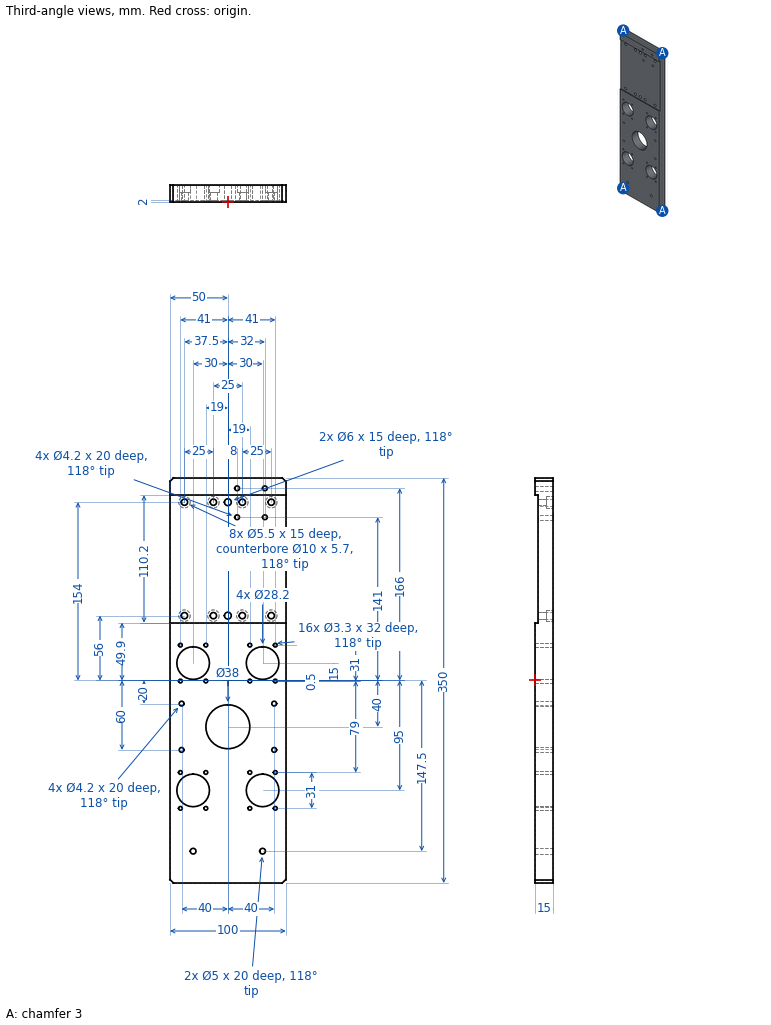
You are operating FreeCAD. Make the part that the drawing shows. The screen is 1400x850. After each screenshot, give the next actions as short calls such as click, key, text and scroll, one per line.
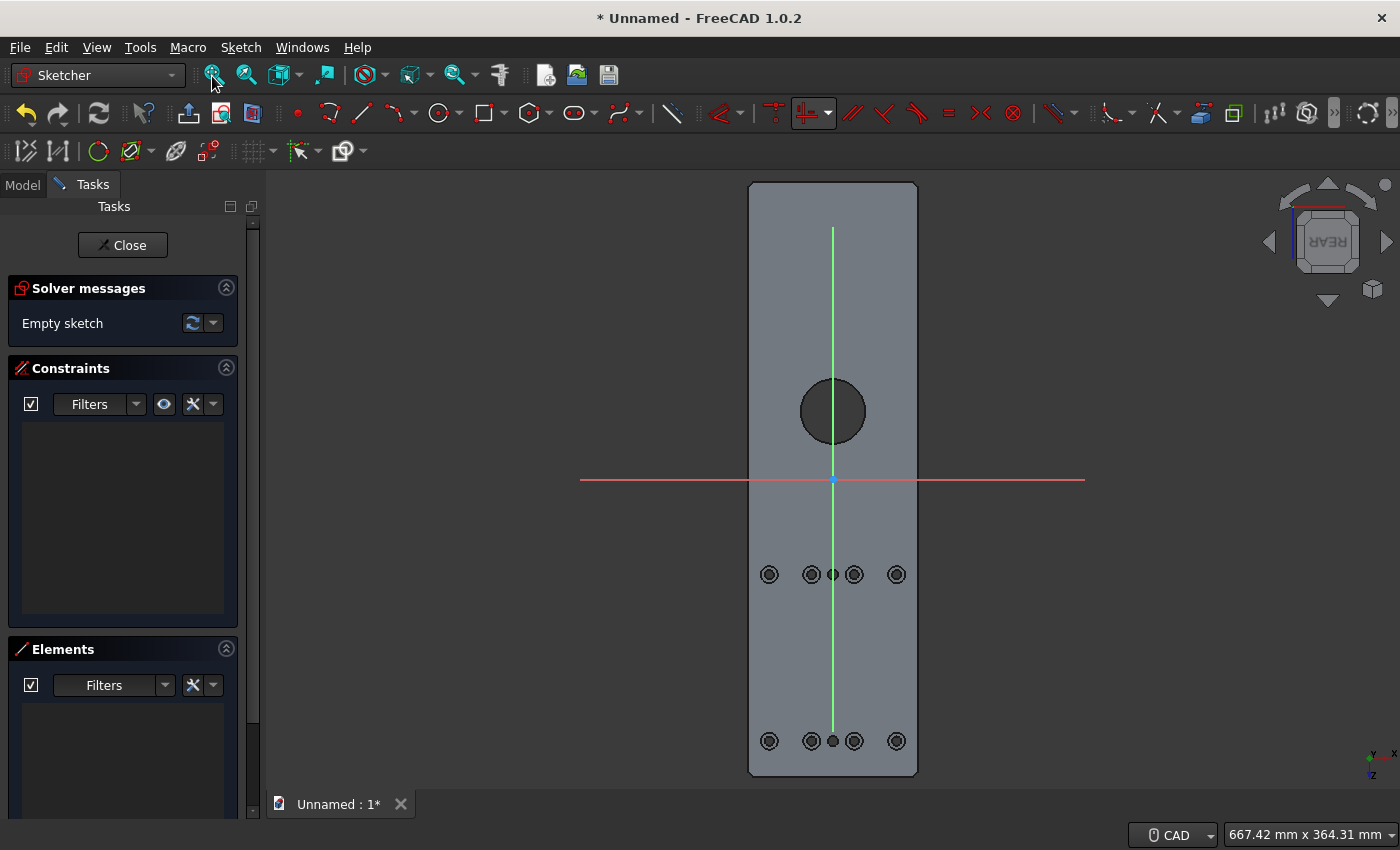
scroll(916, 329, up, 3)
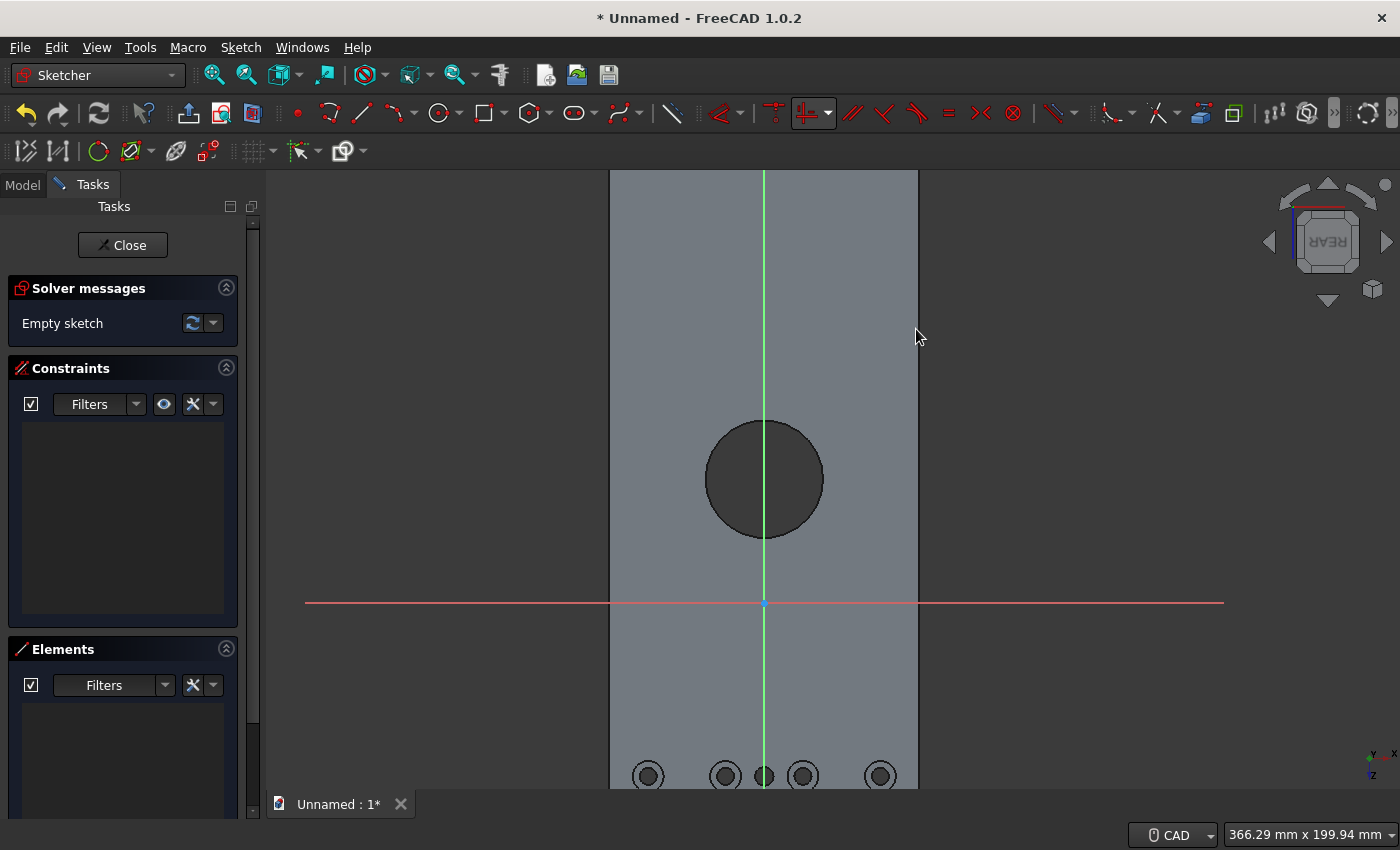
key(g)
key(c)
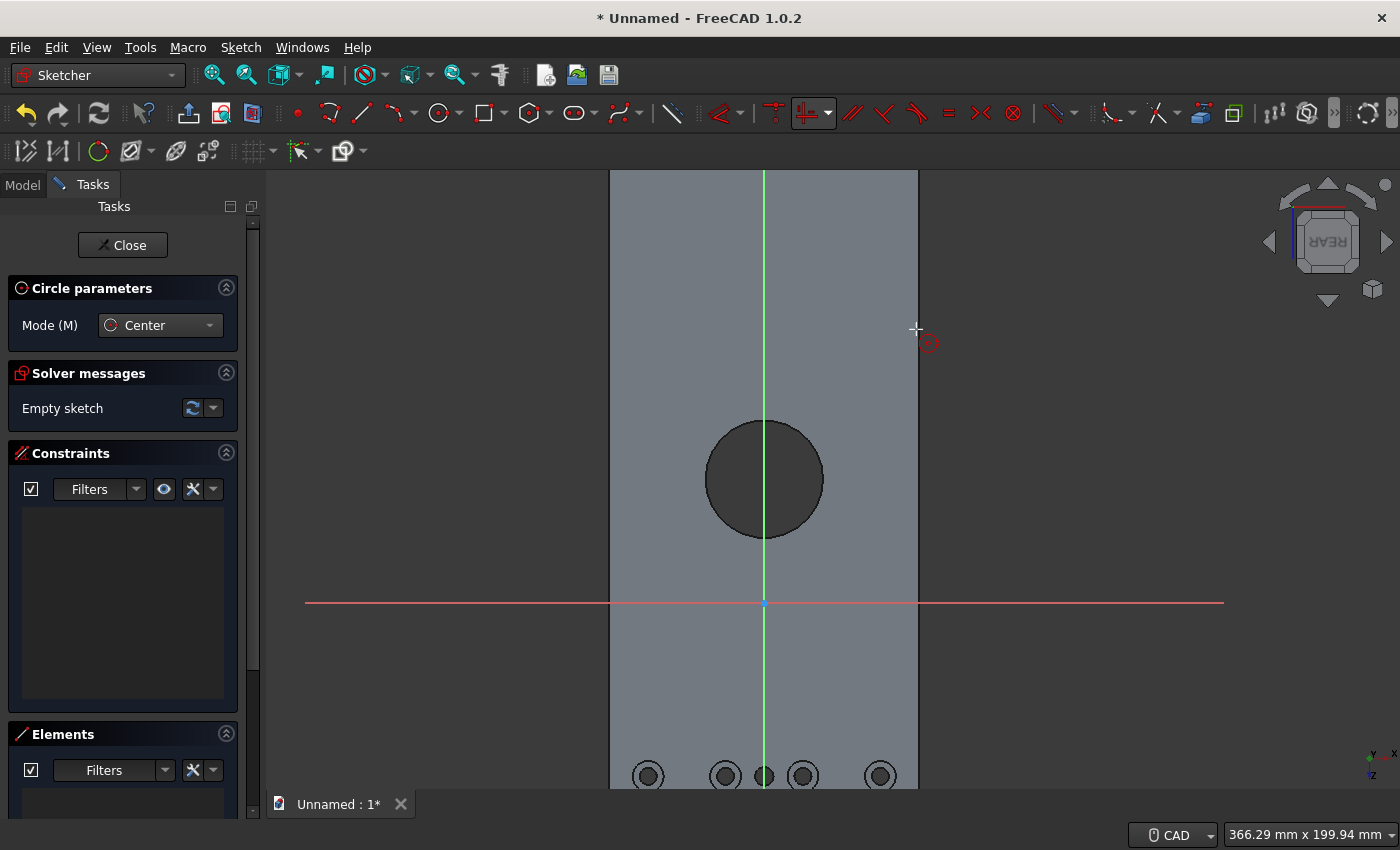
click(857, 649)
click(888, 619)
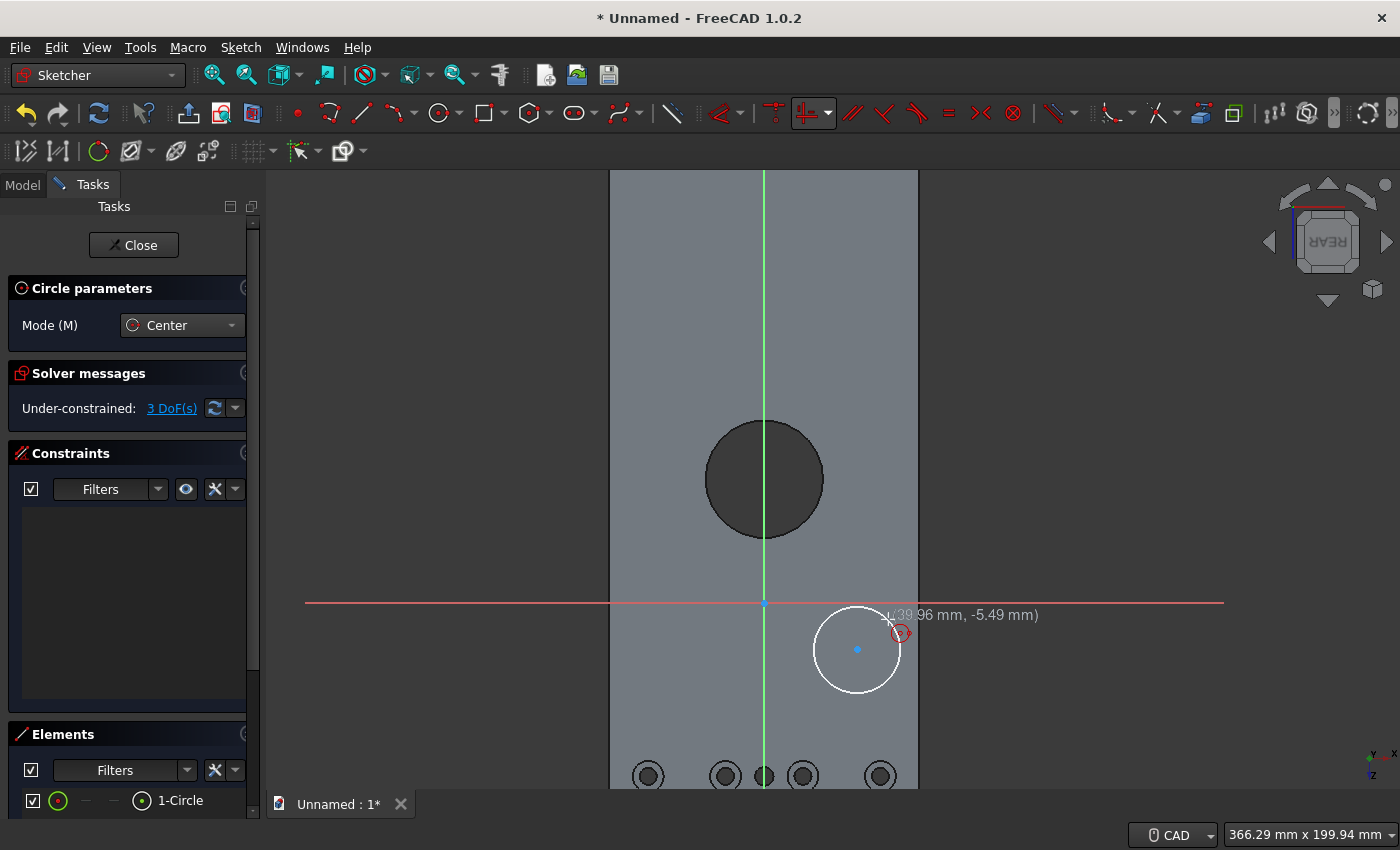
click(857, 309)
click(888, 278)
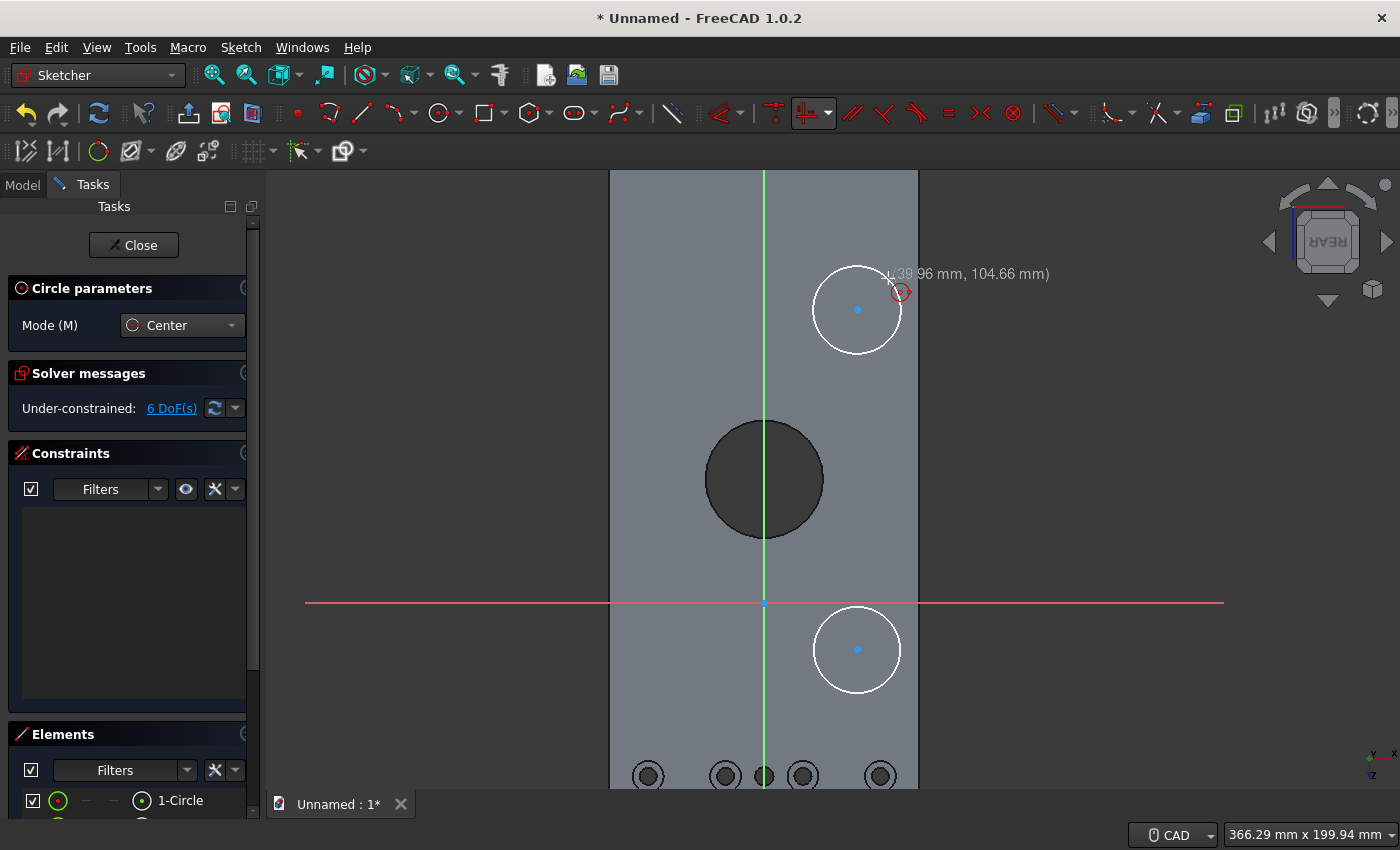
click(671, 649)
click(702, 619)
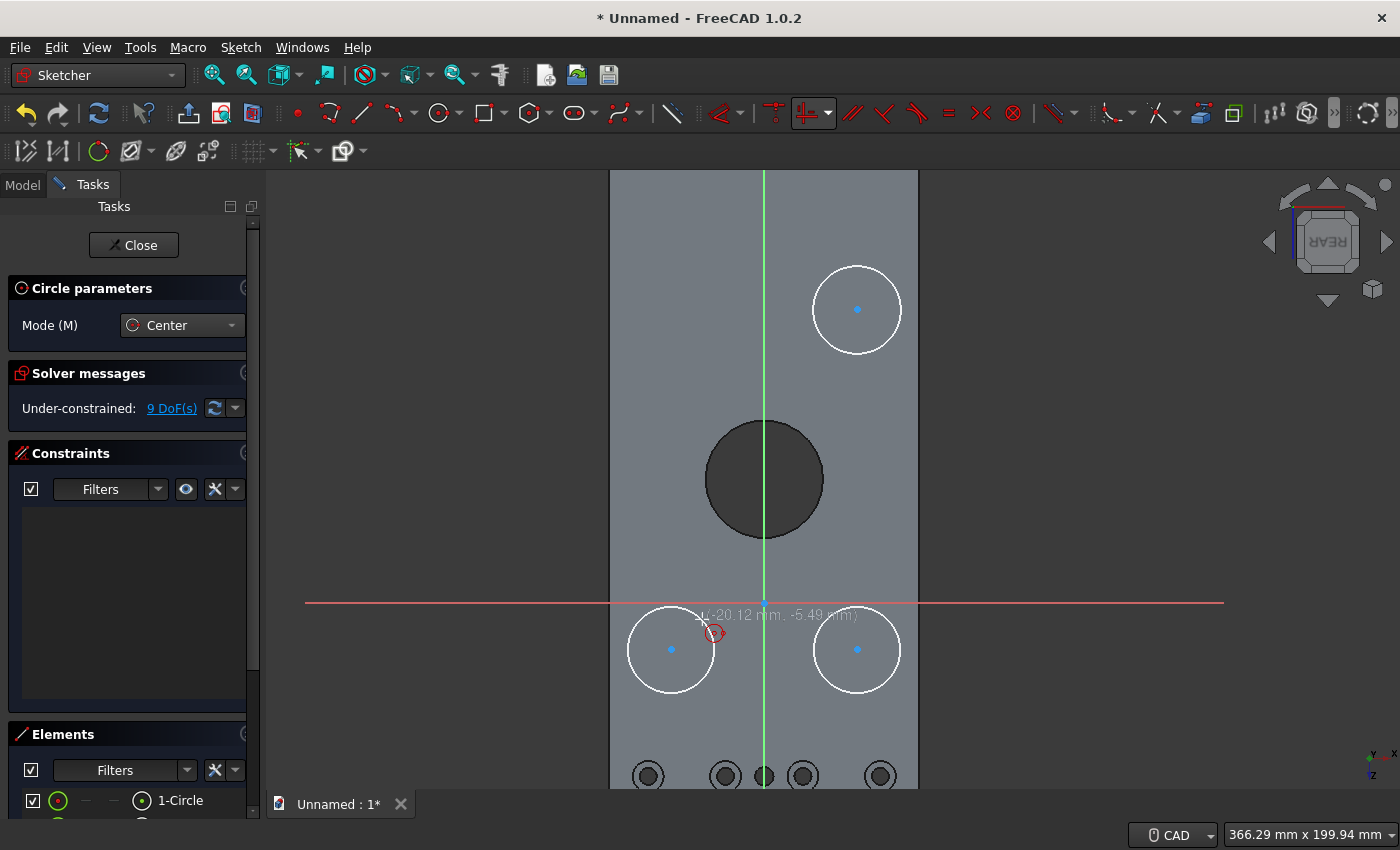
click(671, 309)
click(702, 278)
key(Escape)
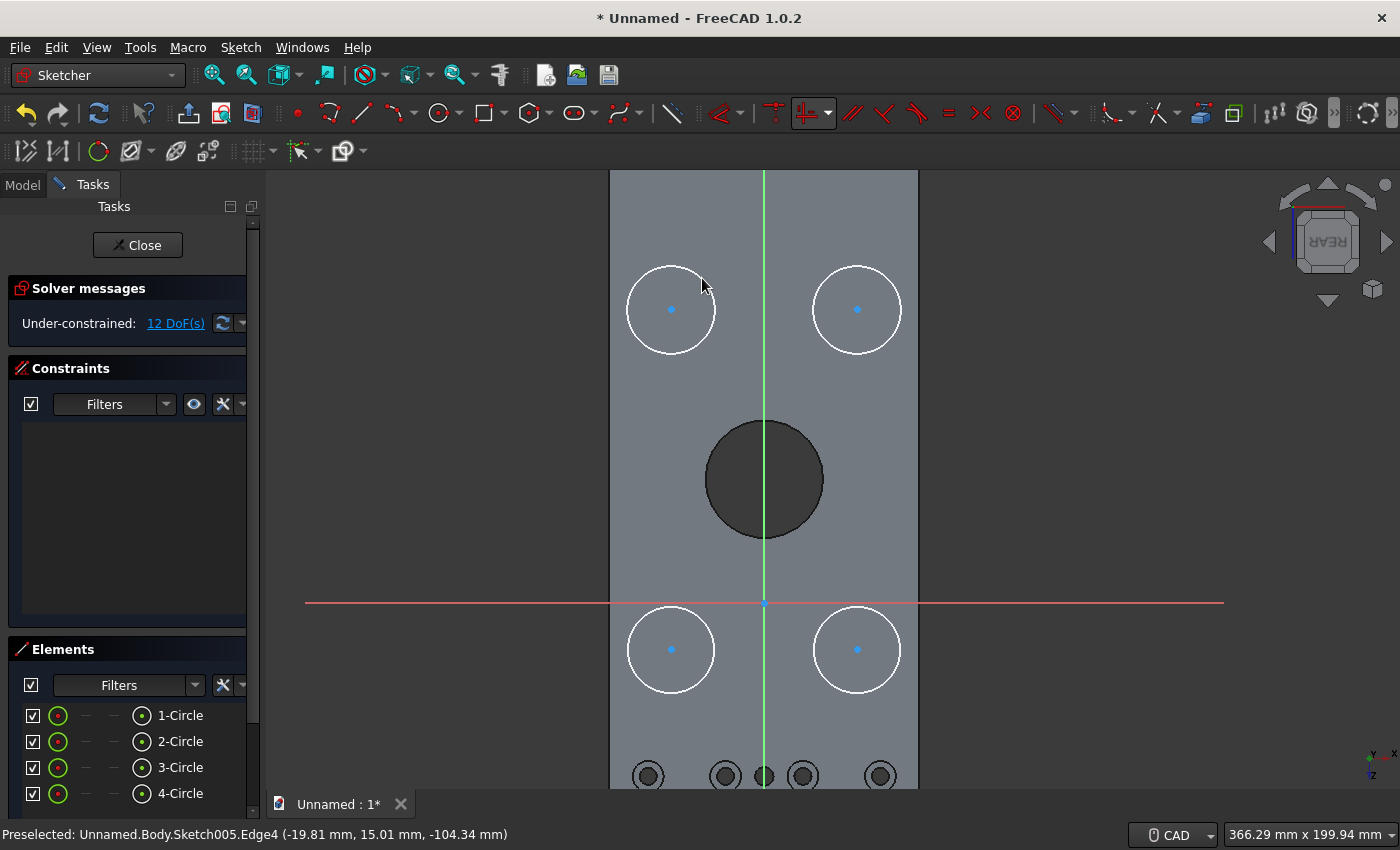
click(887, 619)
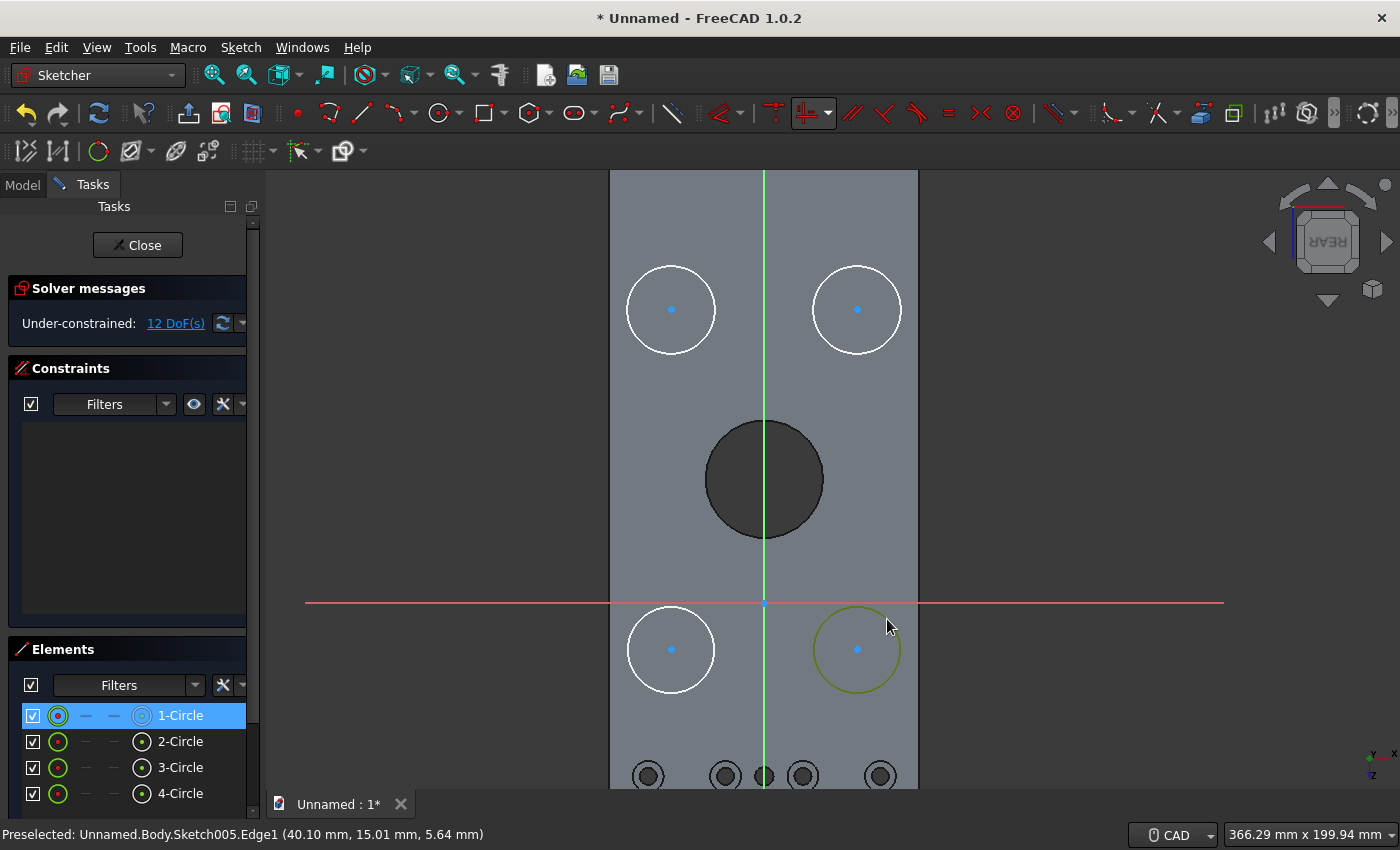
click(888, 279)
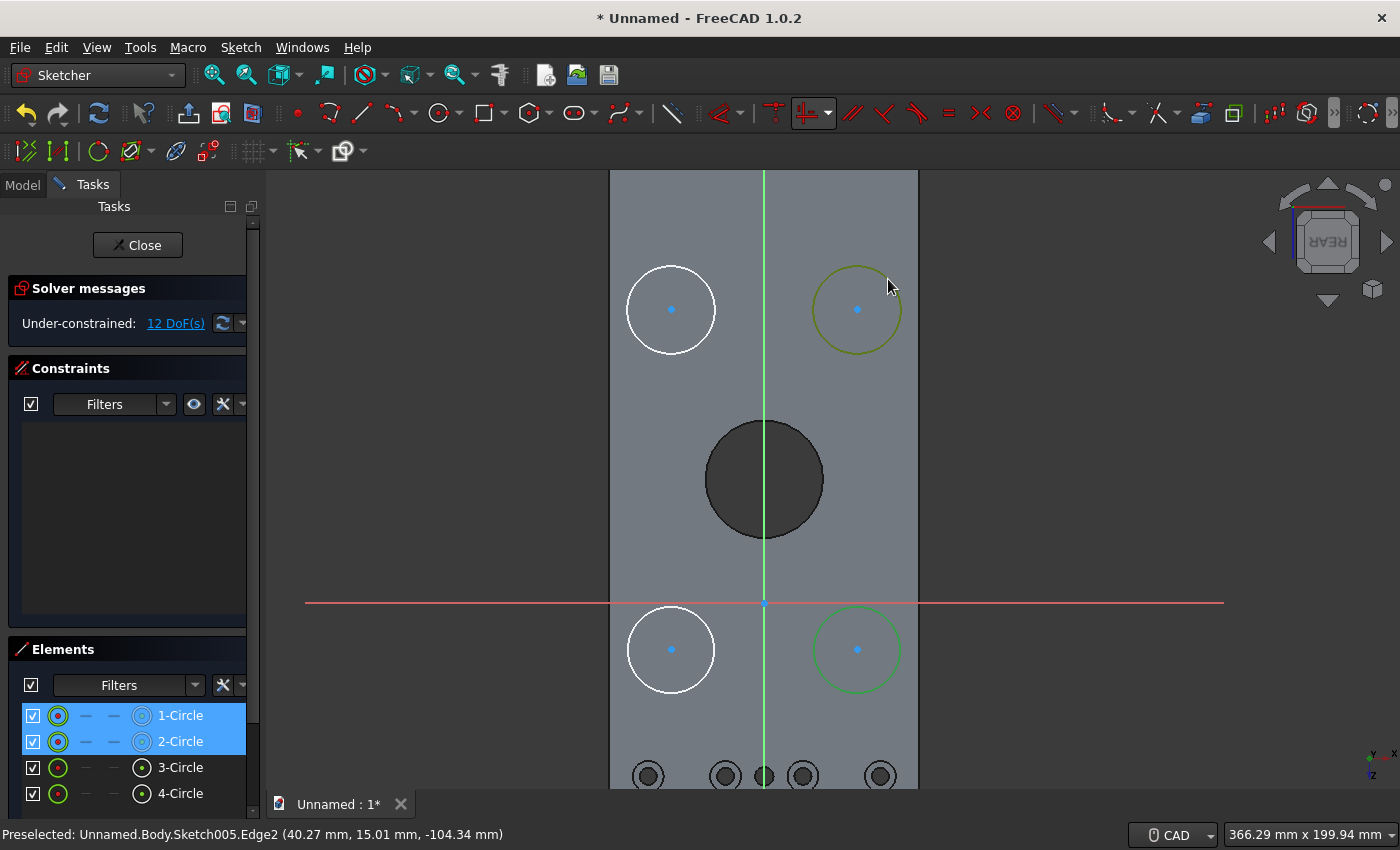
click(701, 619)